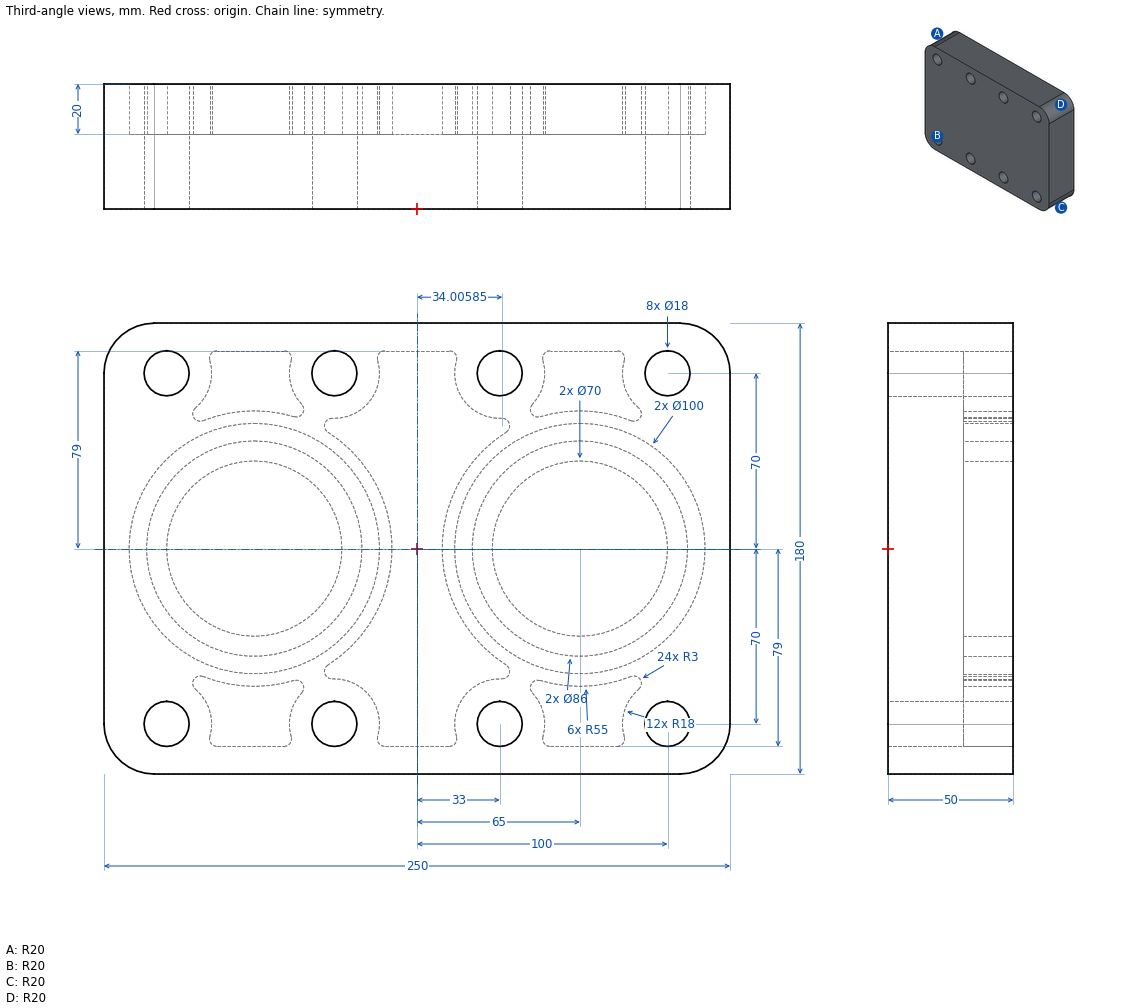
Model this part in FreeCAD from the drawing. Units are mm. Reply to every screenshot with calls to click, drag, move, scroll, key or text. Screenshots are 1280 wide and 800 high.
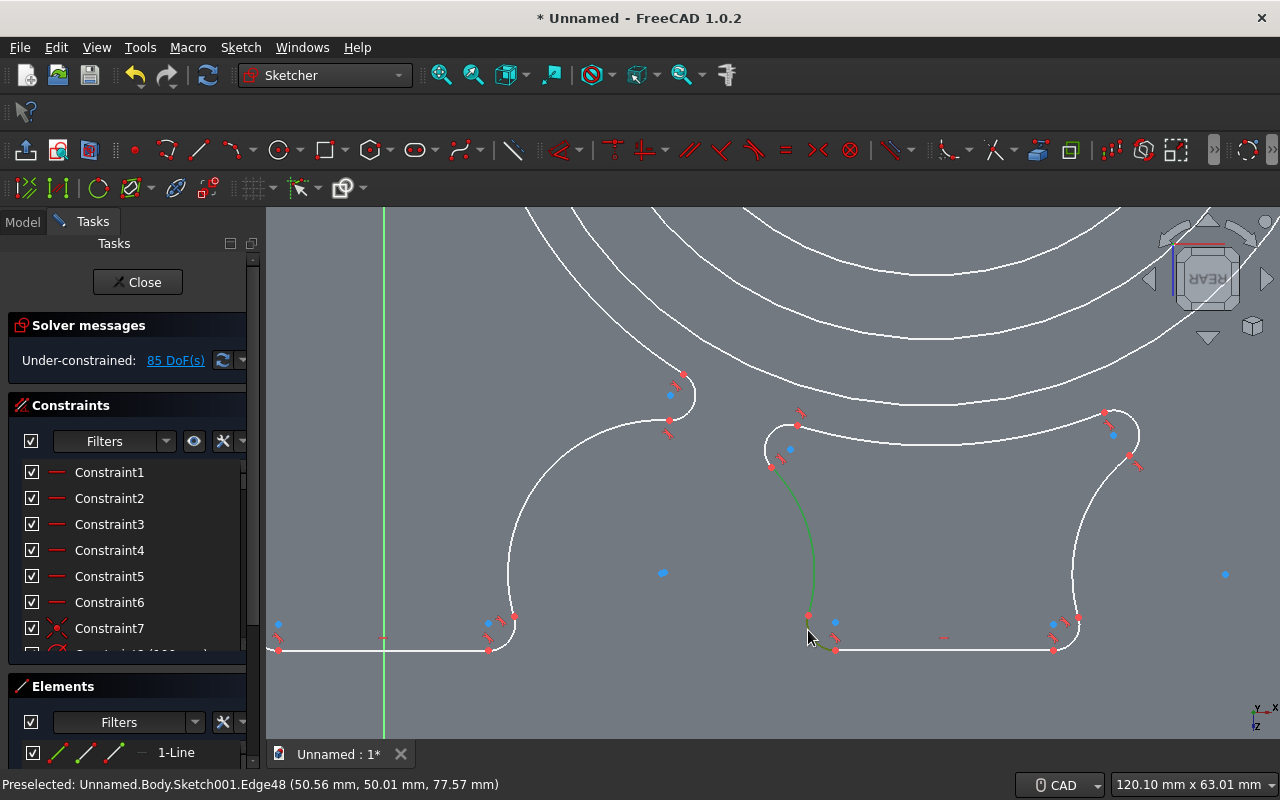
click(754, 150)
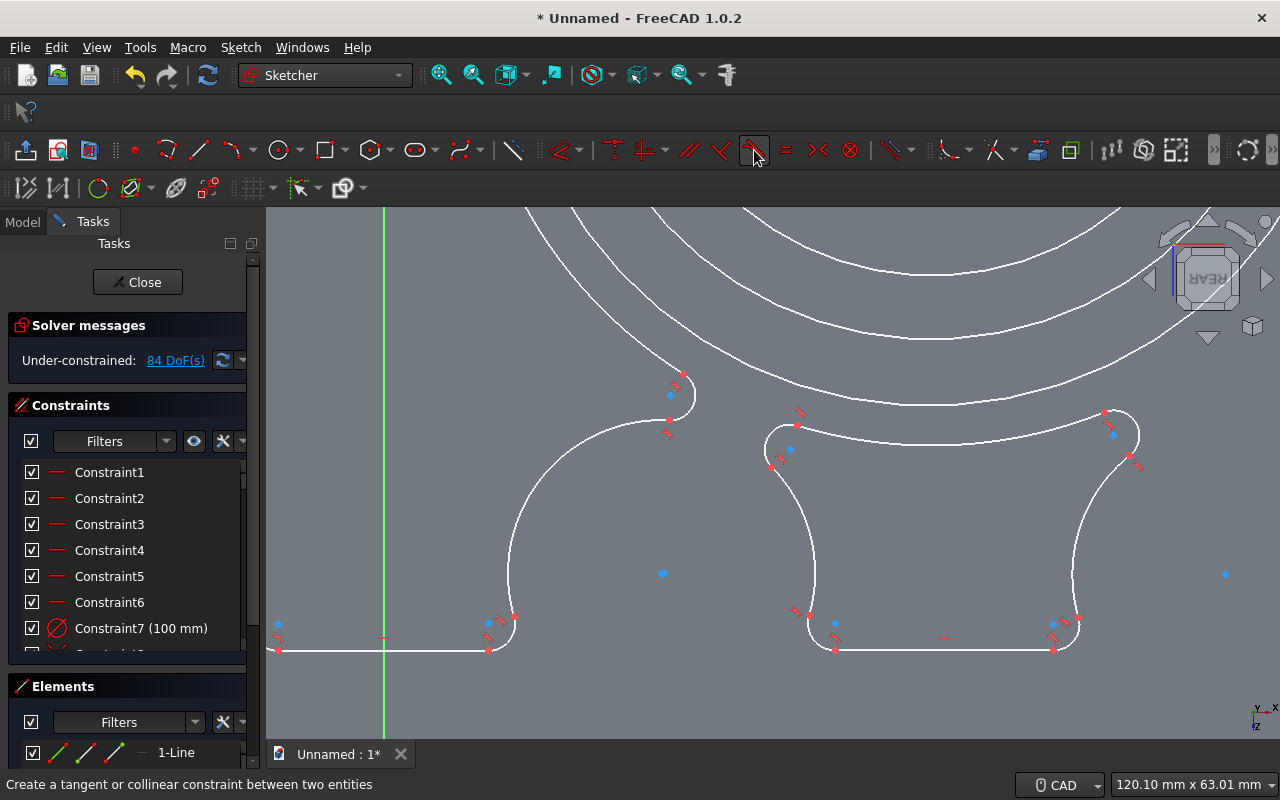
click(631, 283)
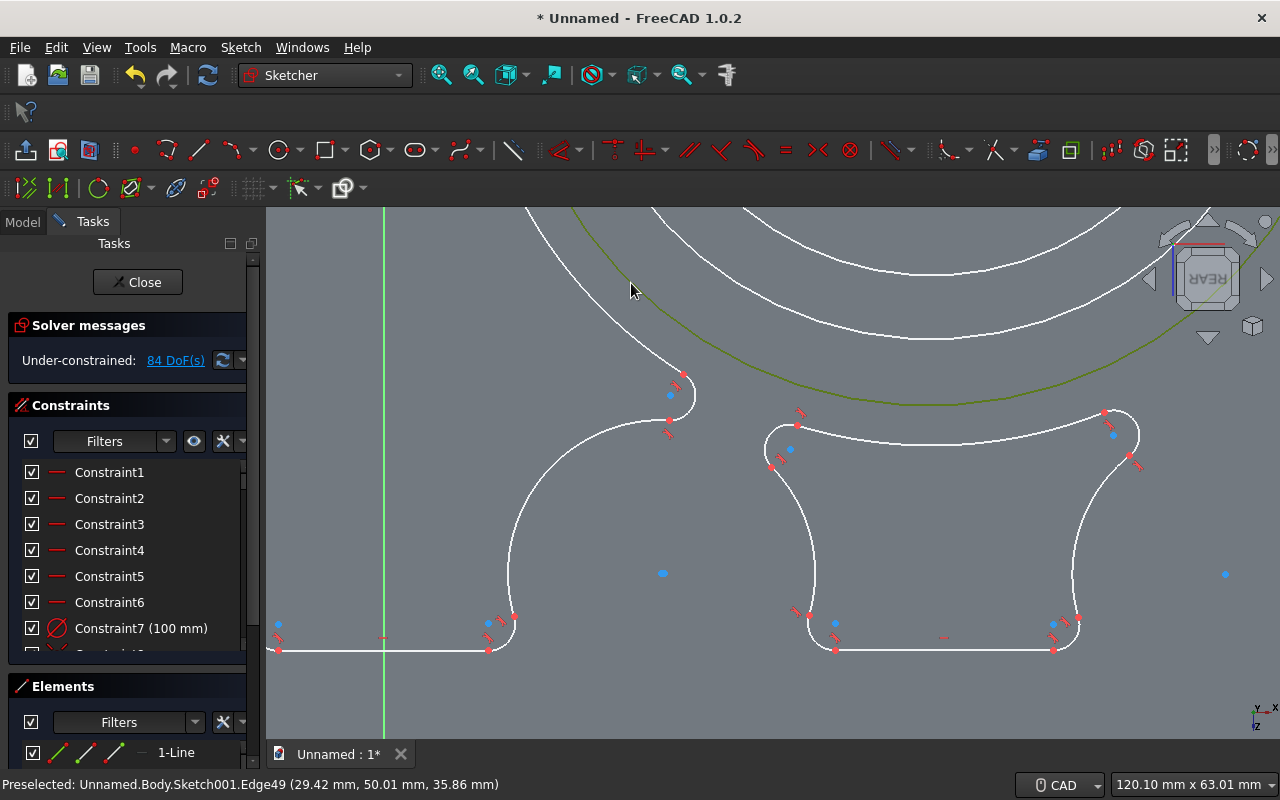
scroll(810, 634, down, 7)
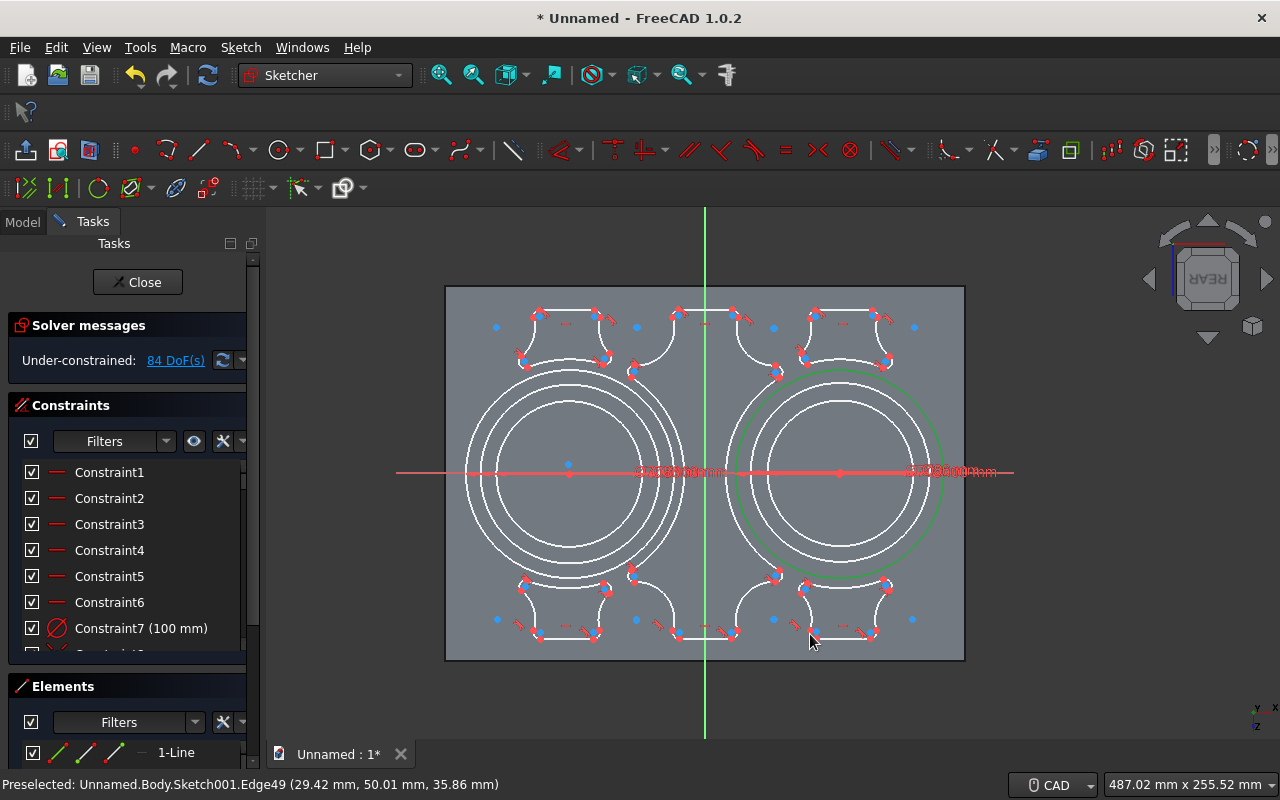
scroll(861, 361, up, 2)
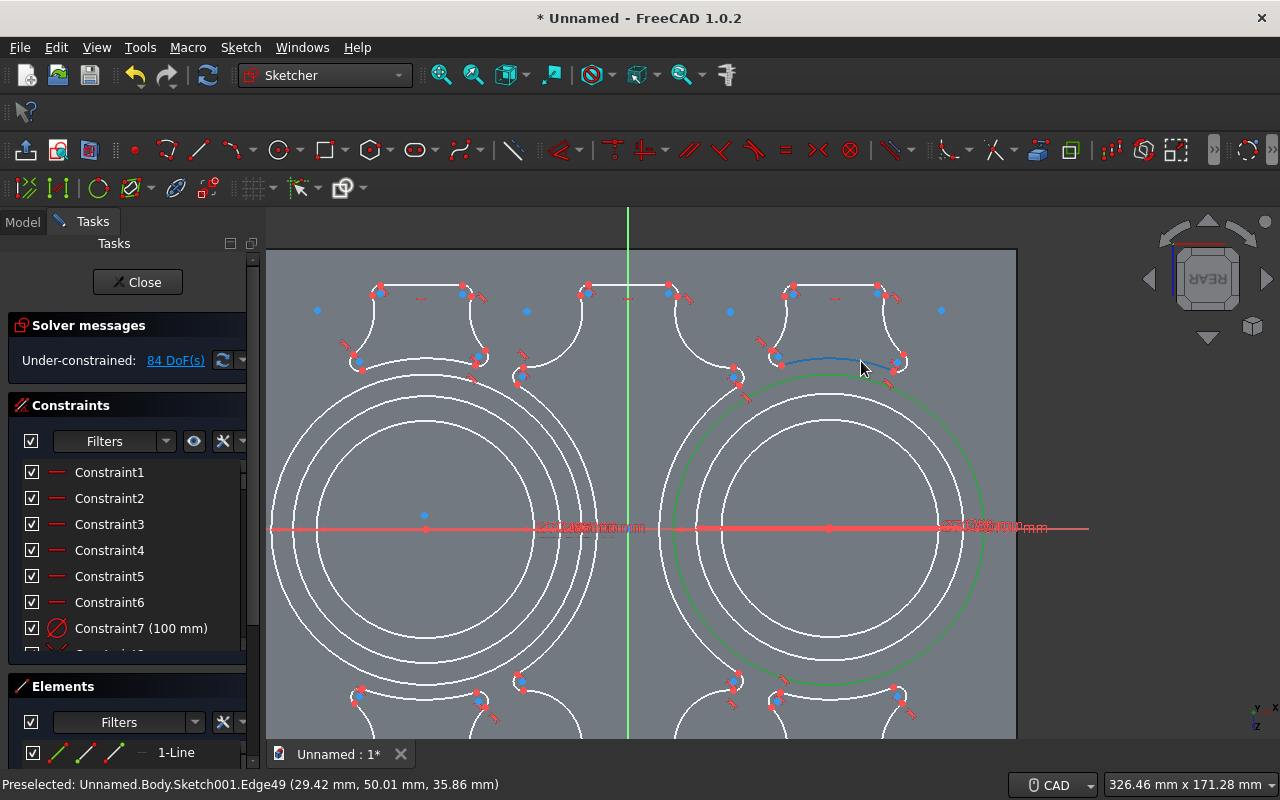
click(861, 361)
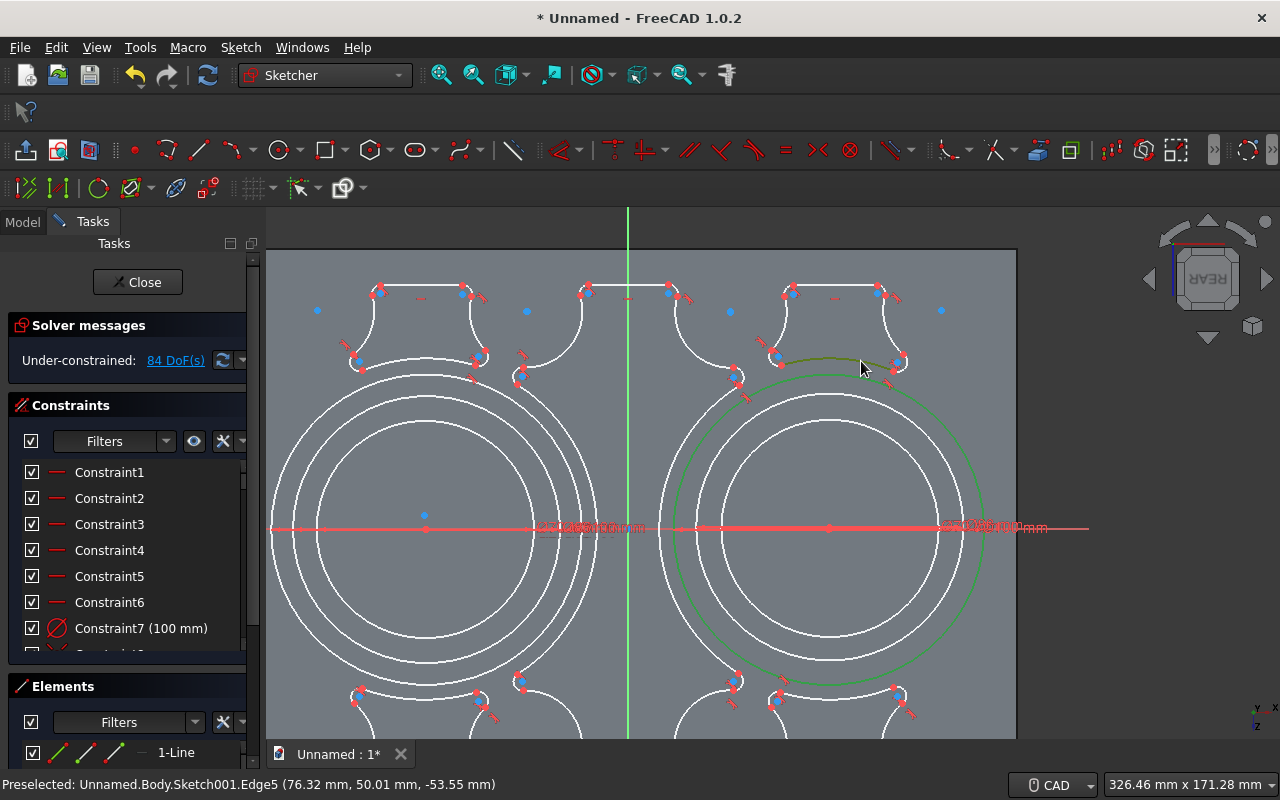
click(614, 150)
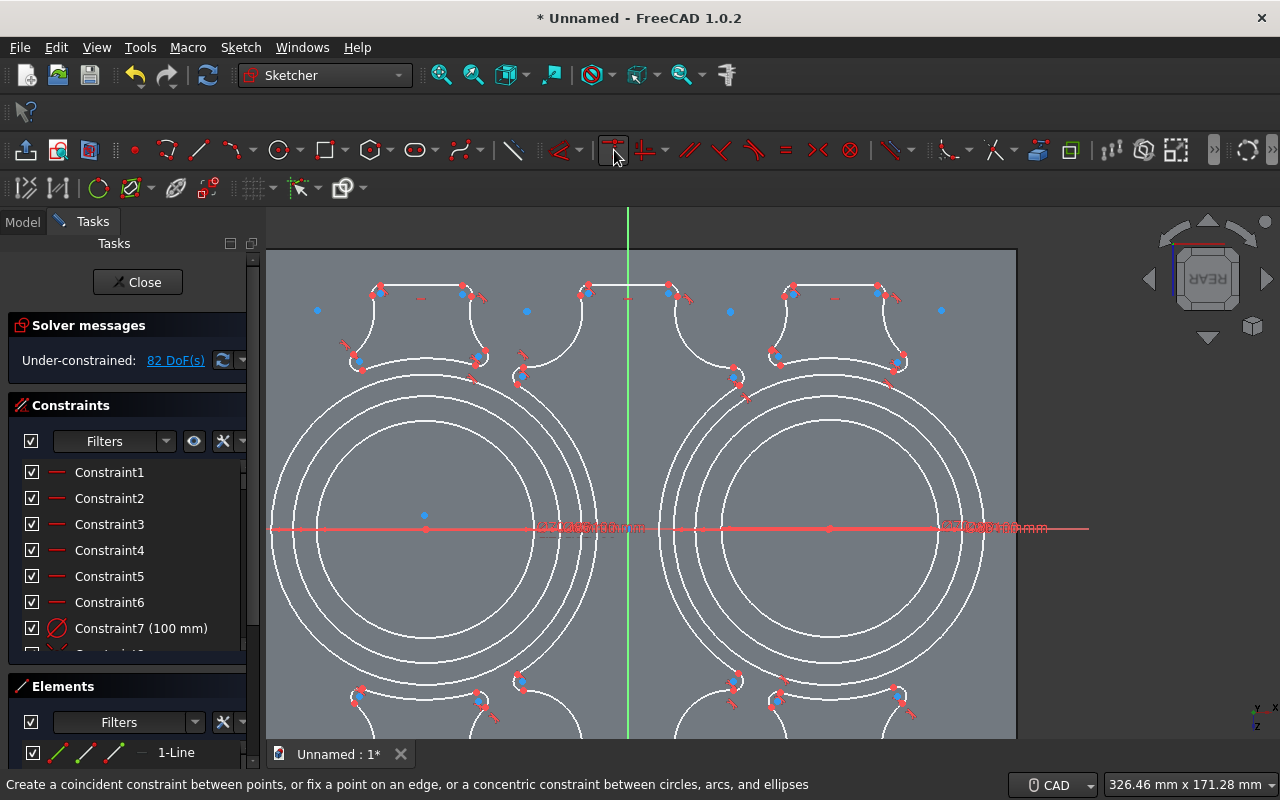
click(781, 336)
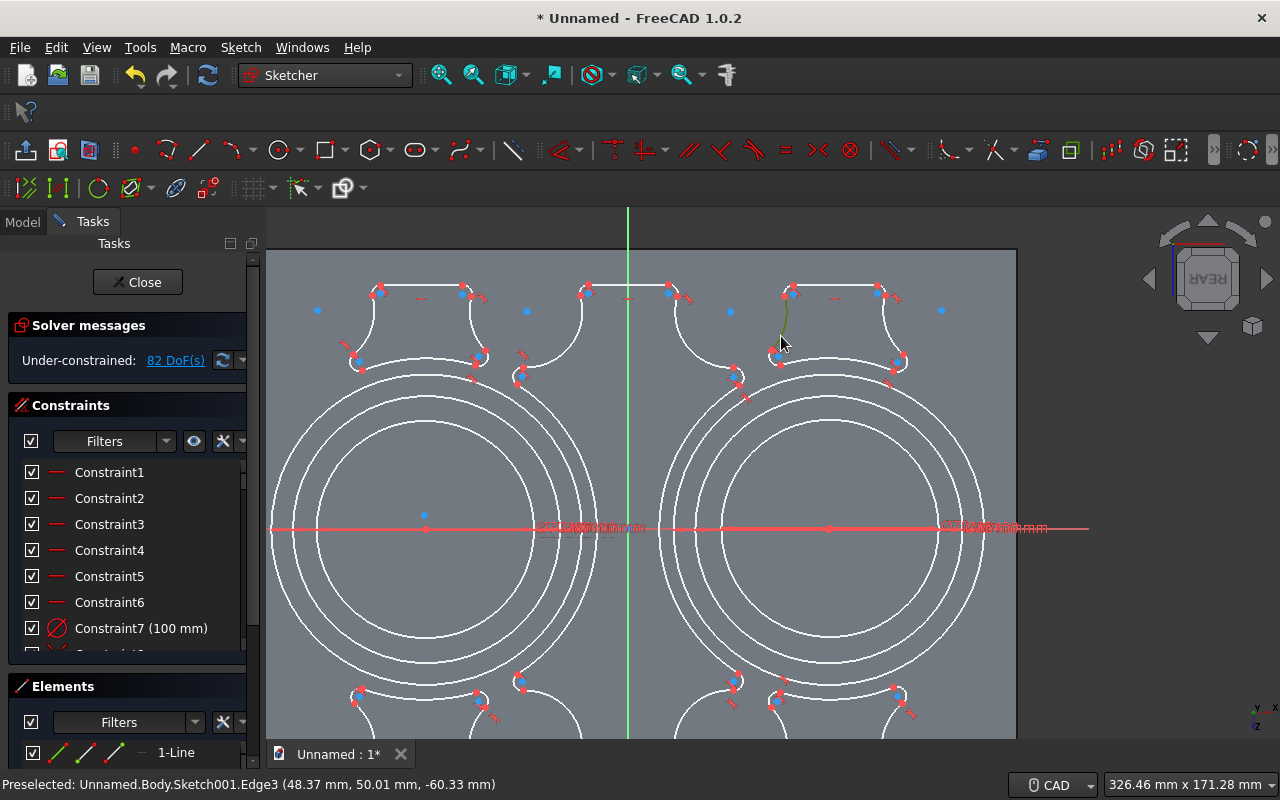
click(677, 328)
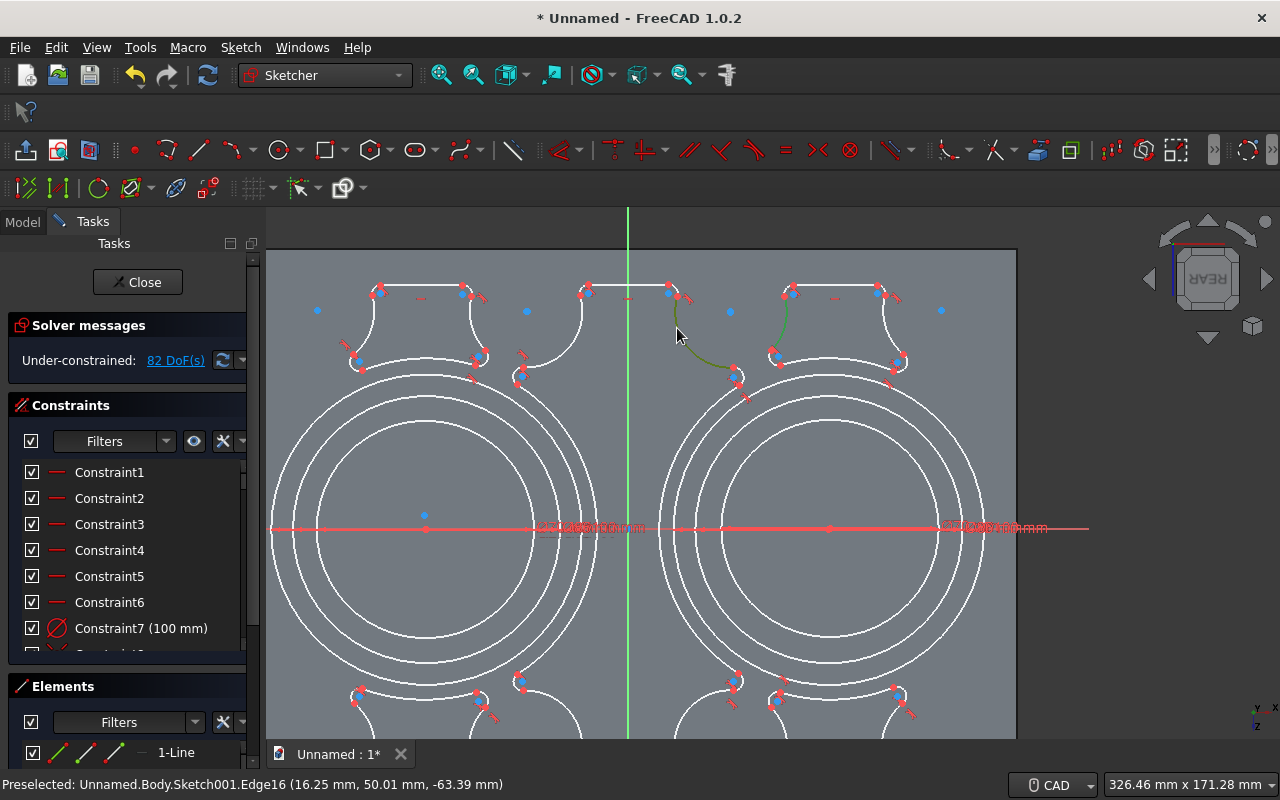
click(614, 150)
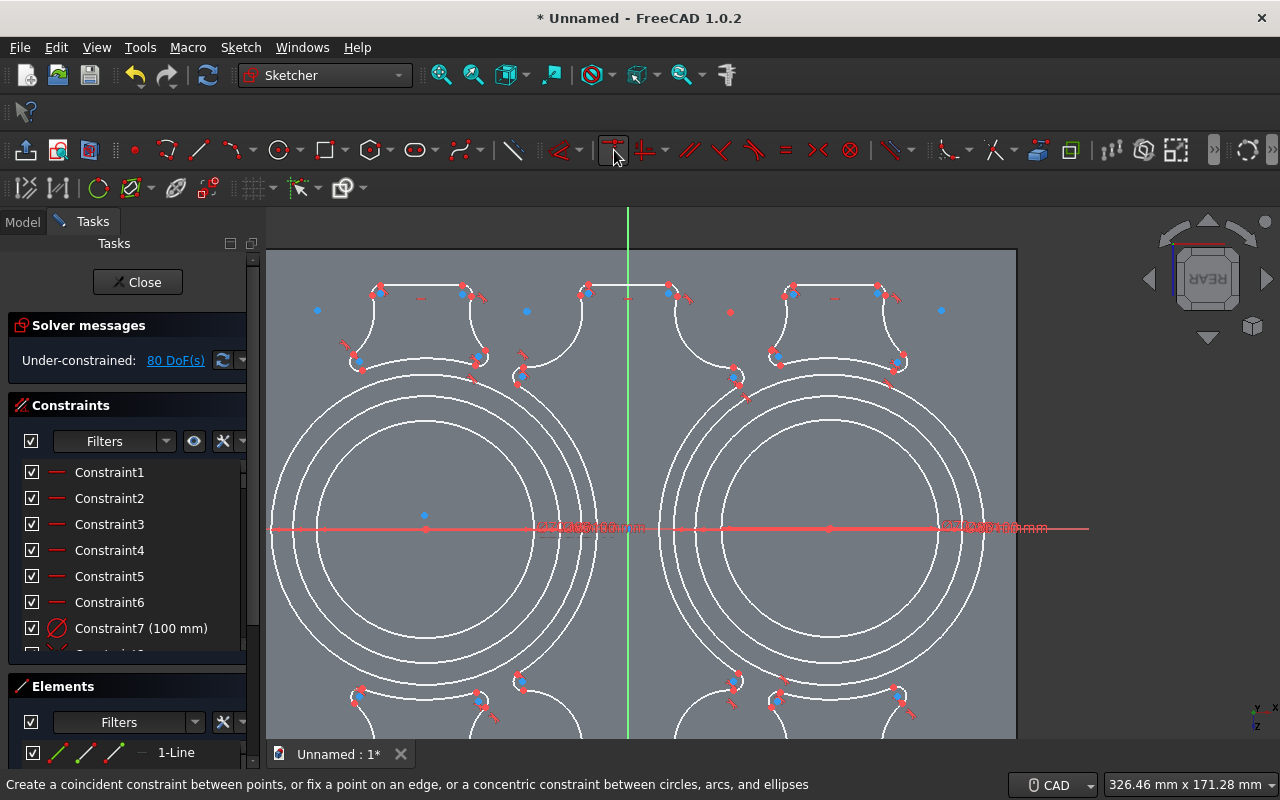
click(536, 419)